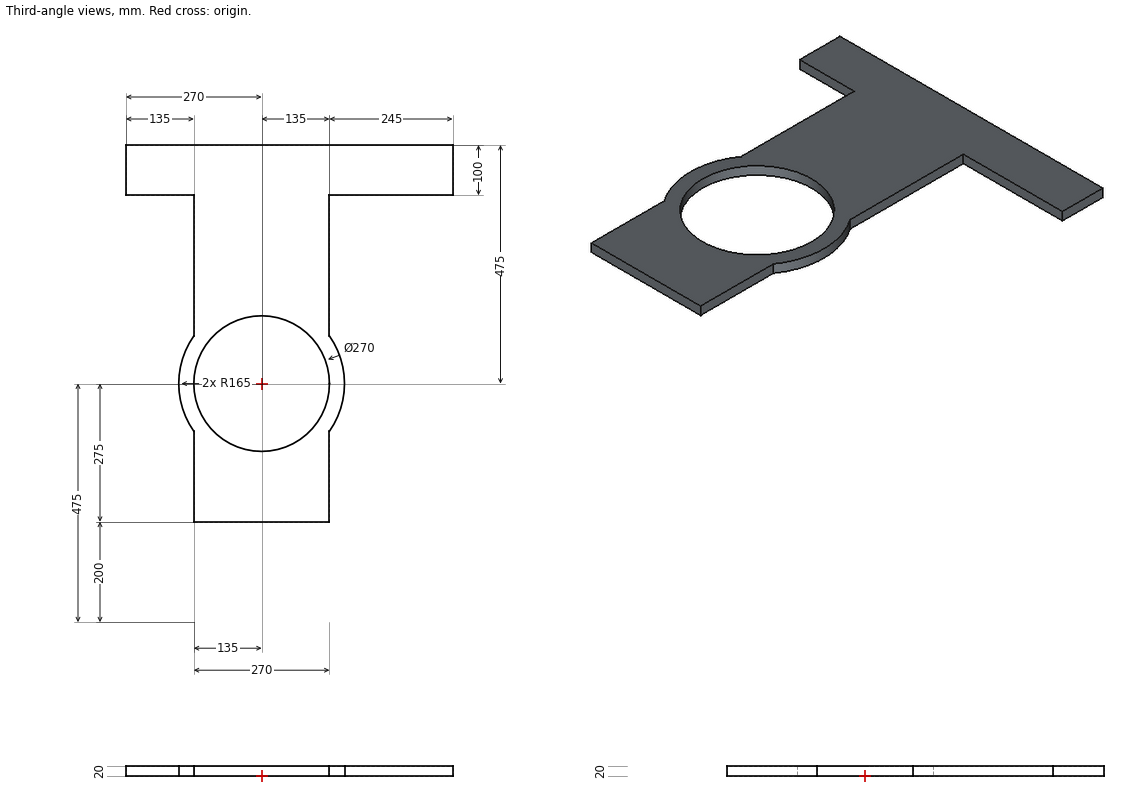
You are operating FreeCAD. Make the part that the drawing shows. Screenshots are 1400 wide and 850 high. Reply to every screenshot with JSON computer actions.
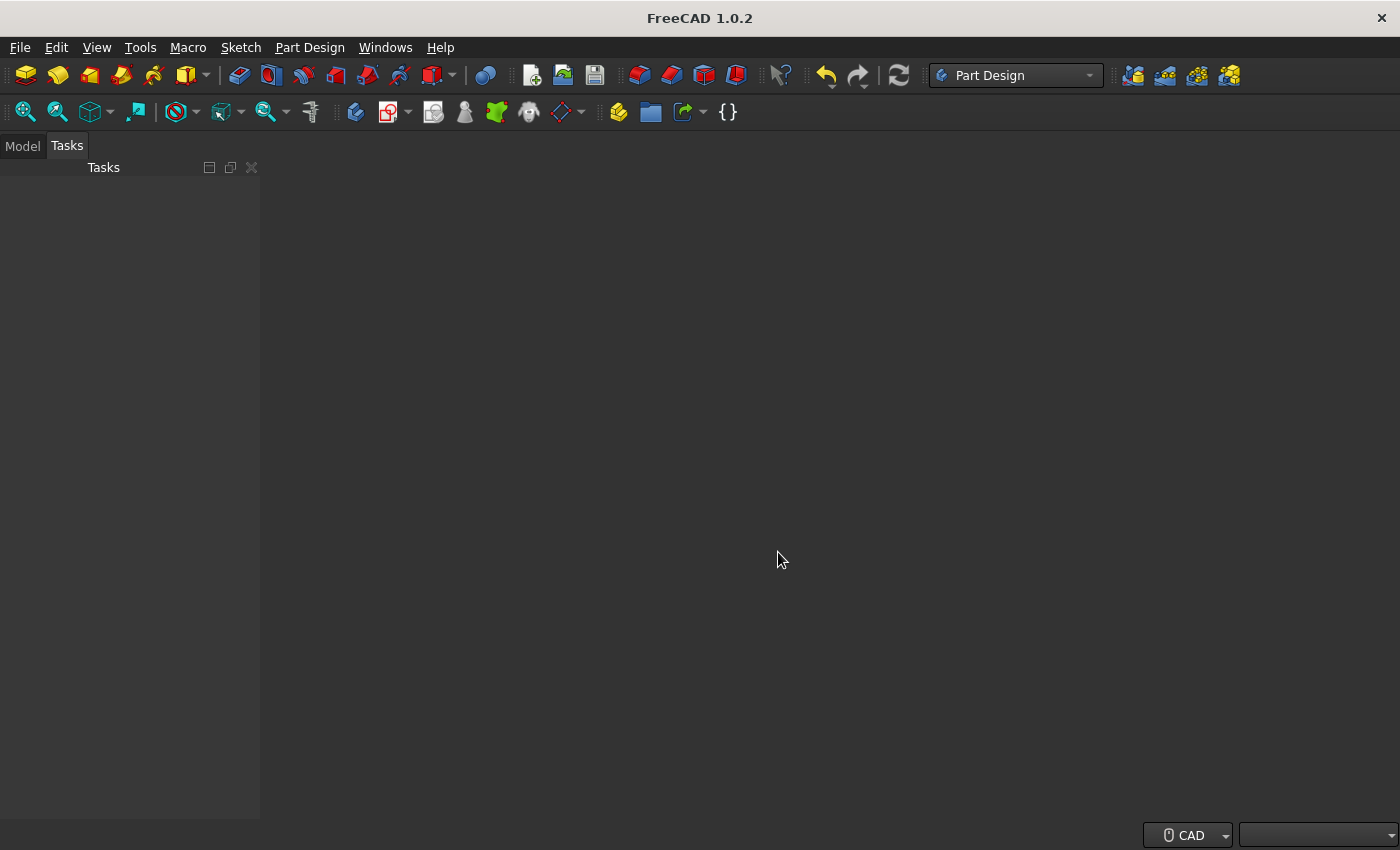
{"action": "key", "text": "ctrl+n"}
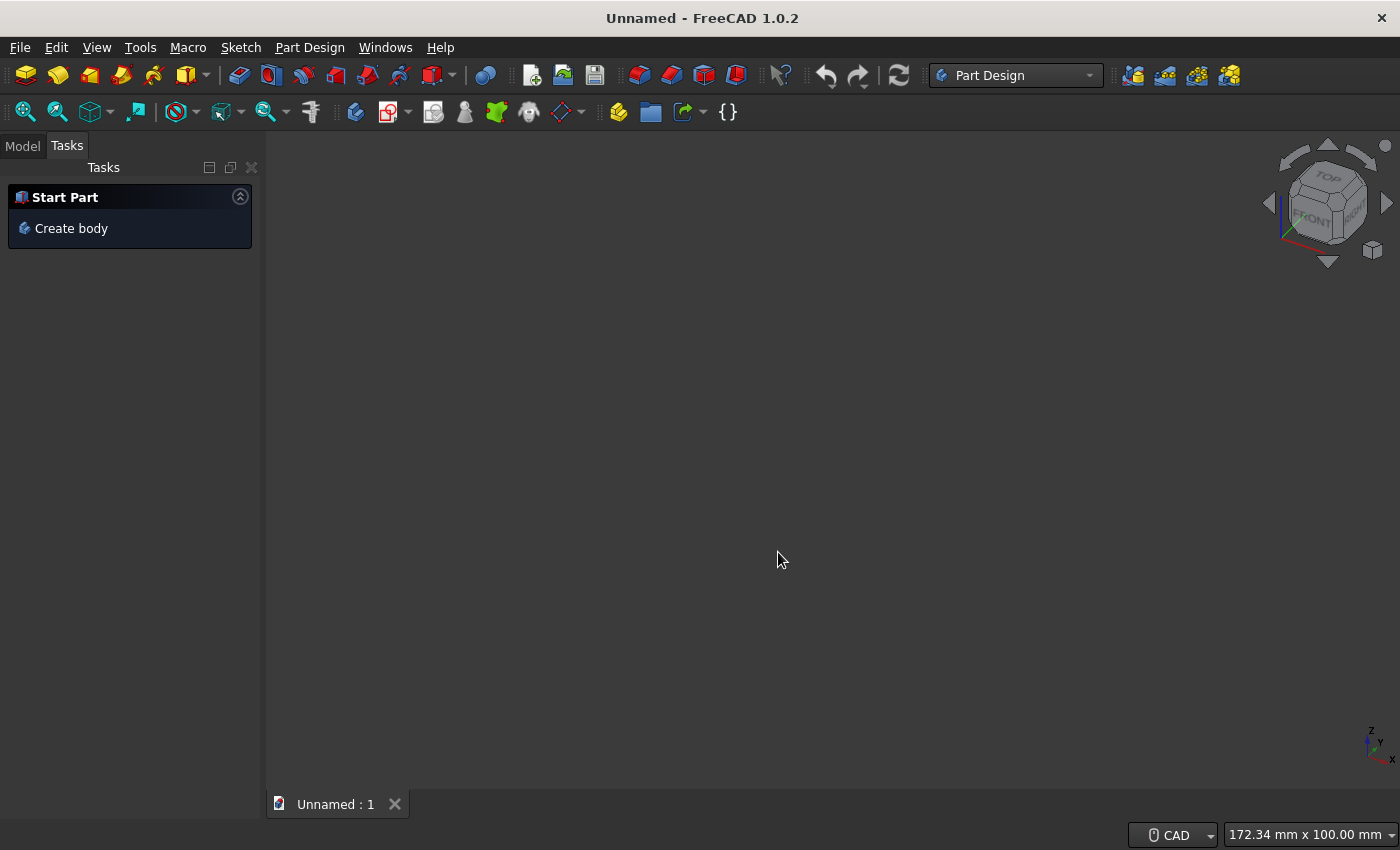
{"action": "left_click", "coordinate": [388, 112]}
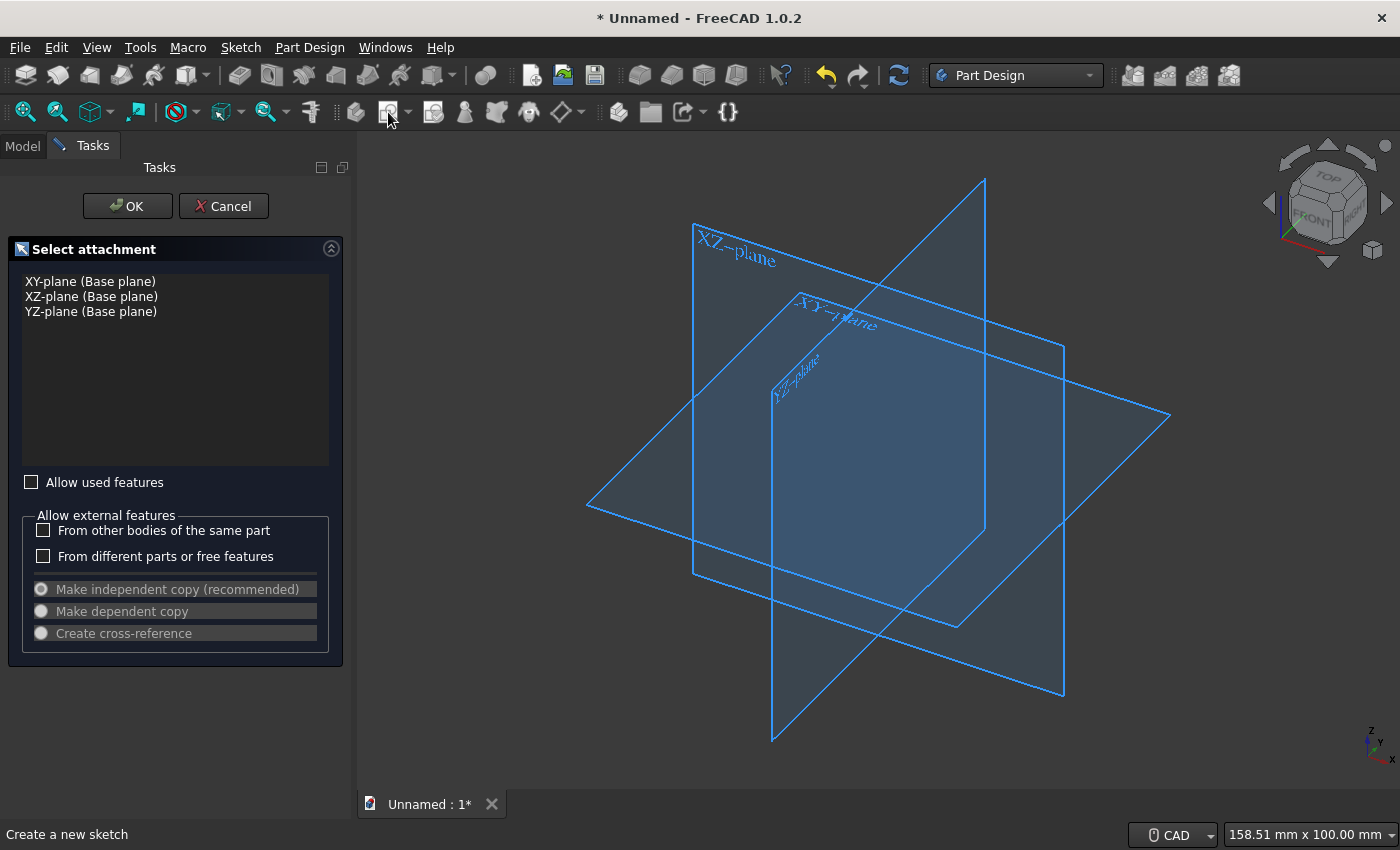
{"action": "left_click", "coordinate": [82, 282]}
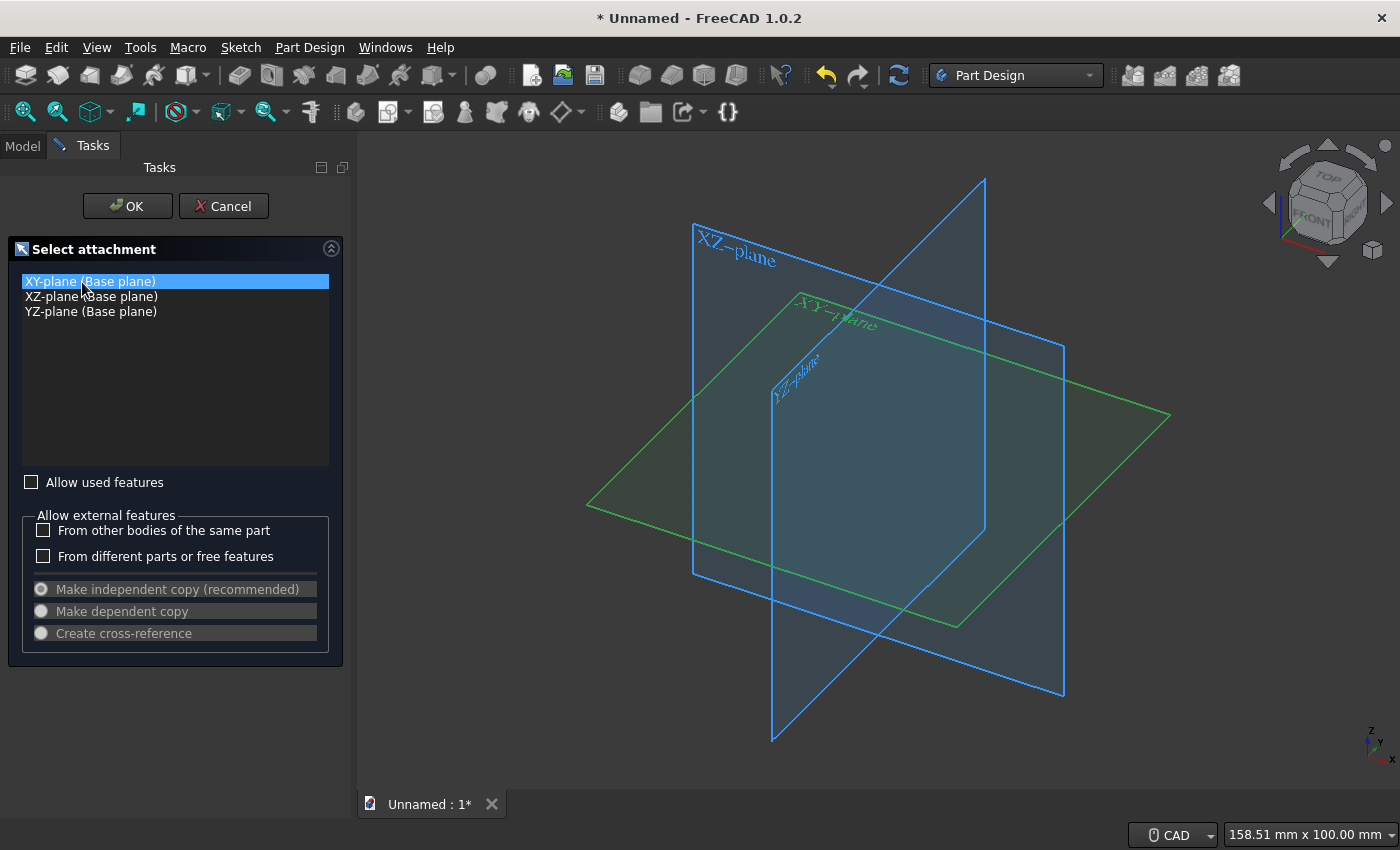
{"action": "left_click", "coordinate": [128, 206]}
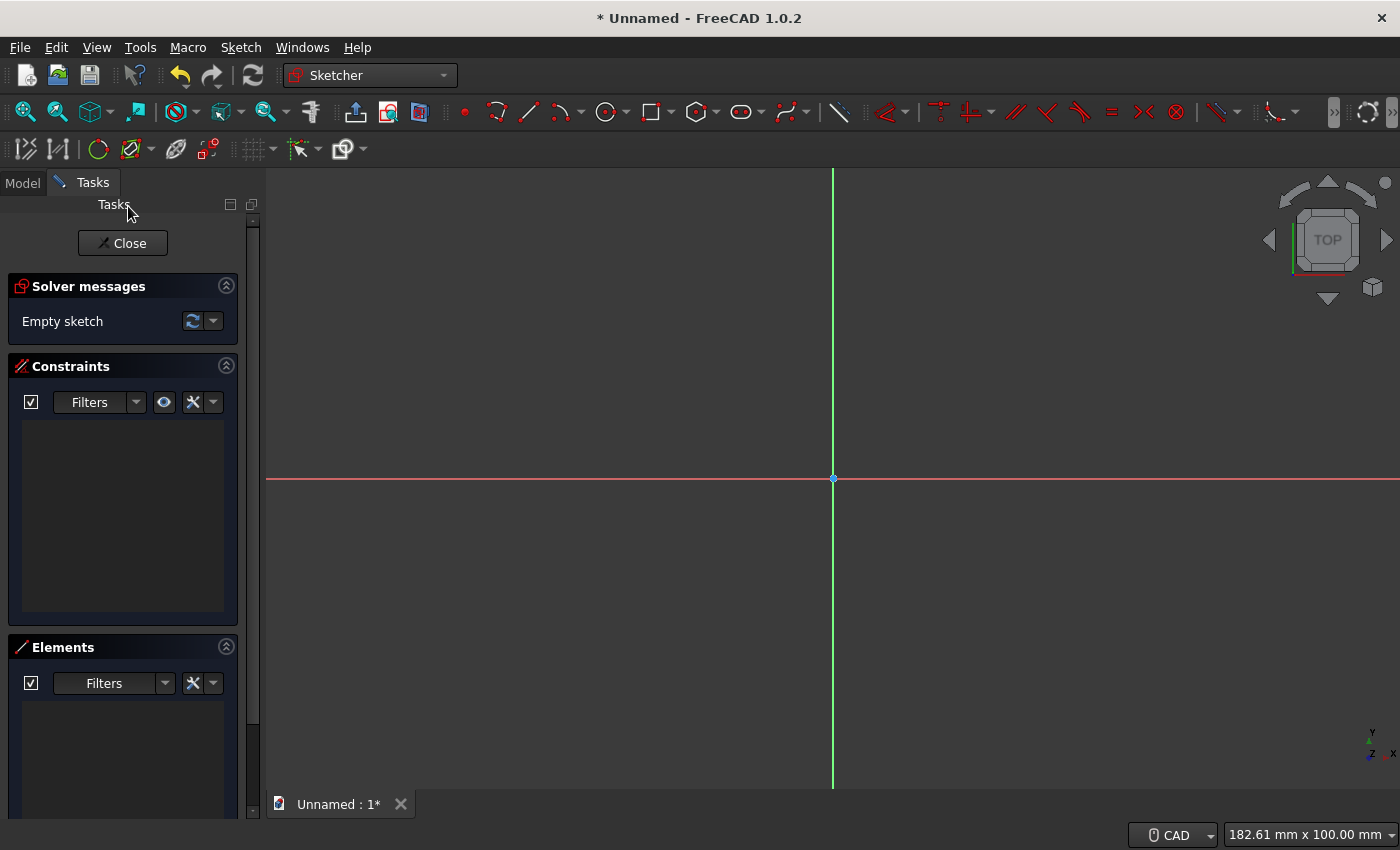
{"action": "scroll", "coordinate": [759, 478], "scroll_direction": "down", "scroll_amount": 13}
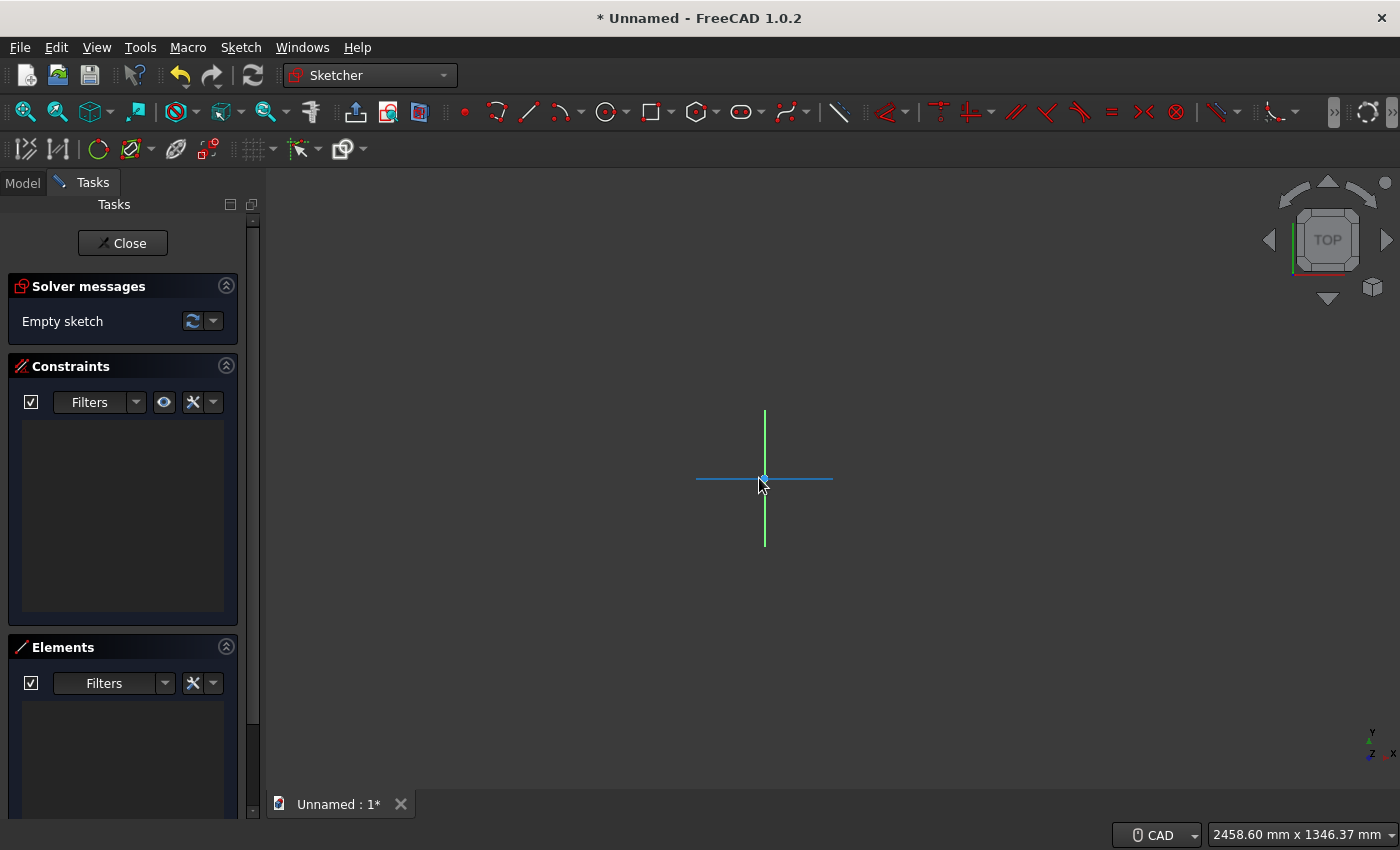
{"action": "key", "text": "g m"}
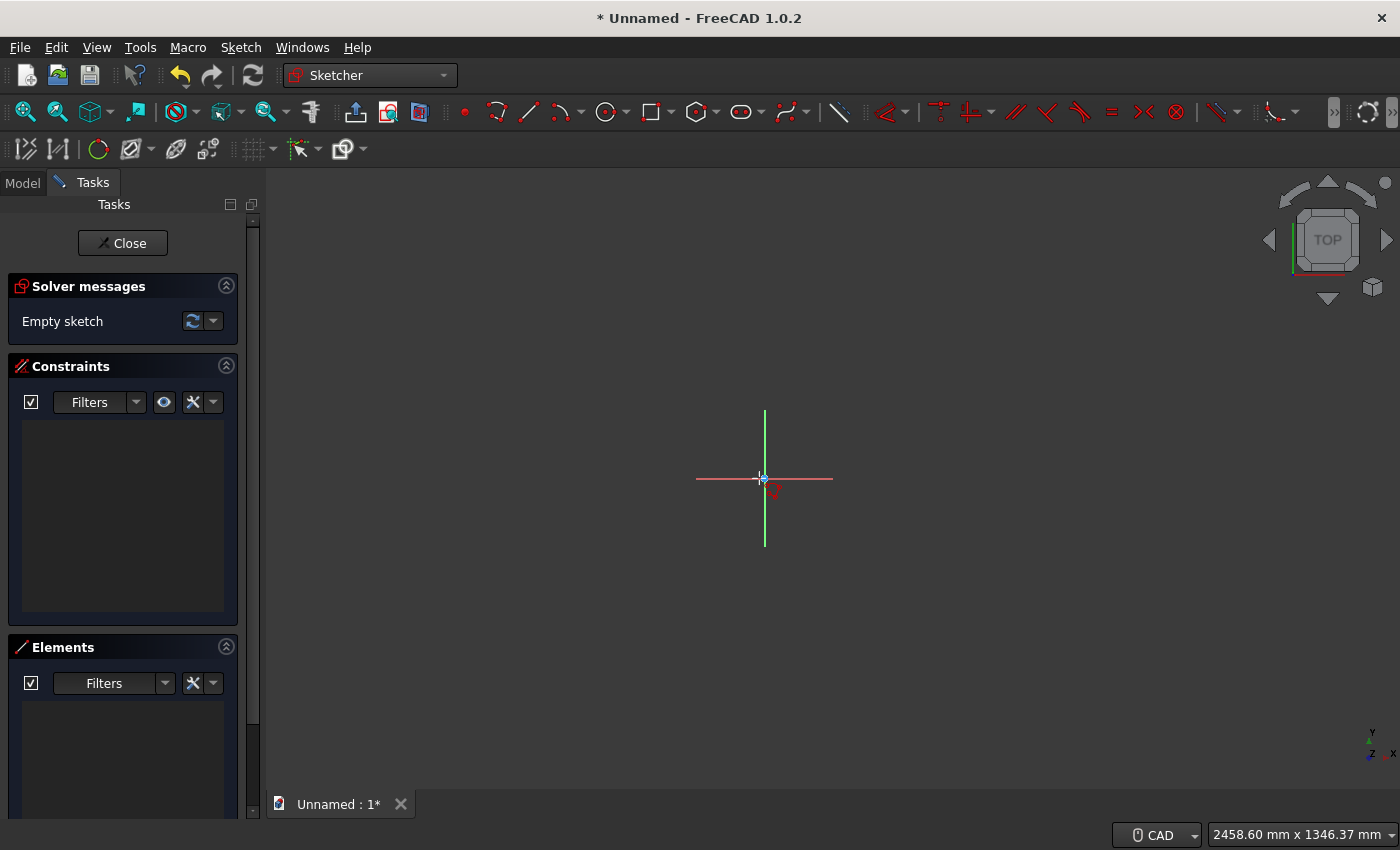
{"action": "left_click", "coordinate": [703, 522]}
{"action": "left_click", "coordinate": [703, 698]}
{"action": "left_click", "coordinate": [827, 698]}
{"action": "left_click", "coordinate": [827, 522]}
{"action": "right_click", "coordinate": [827, 522]}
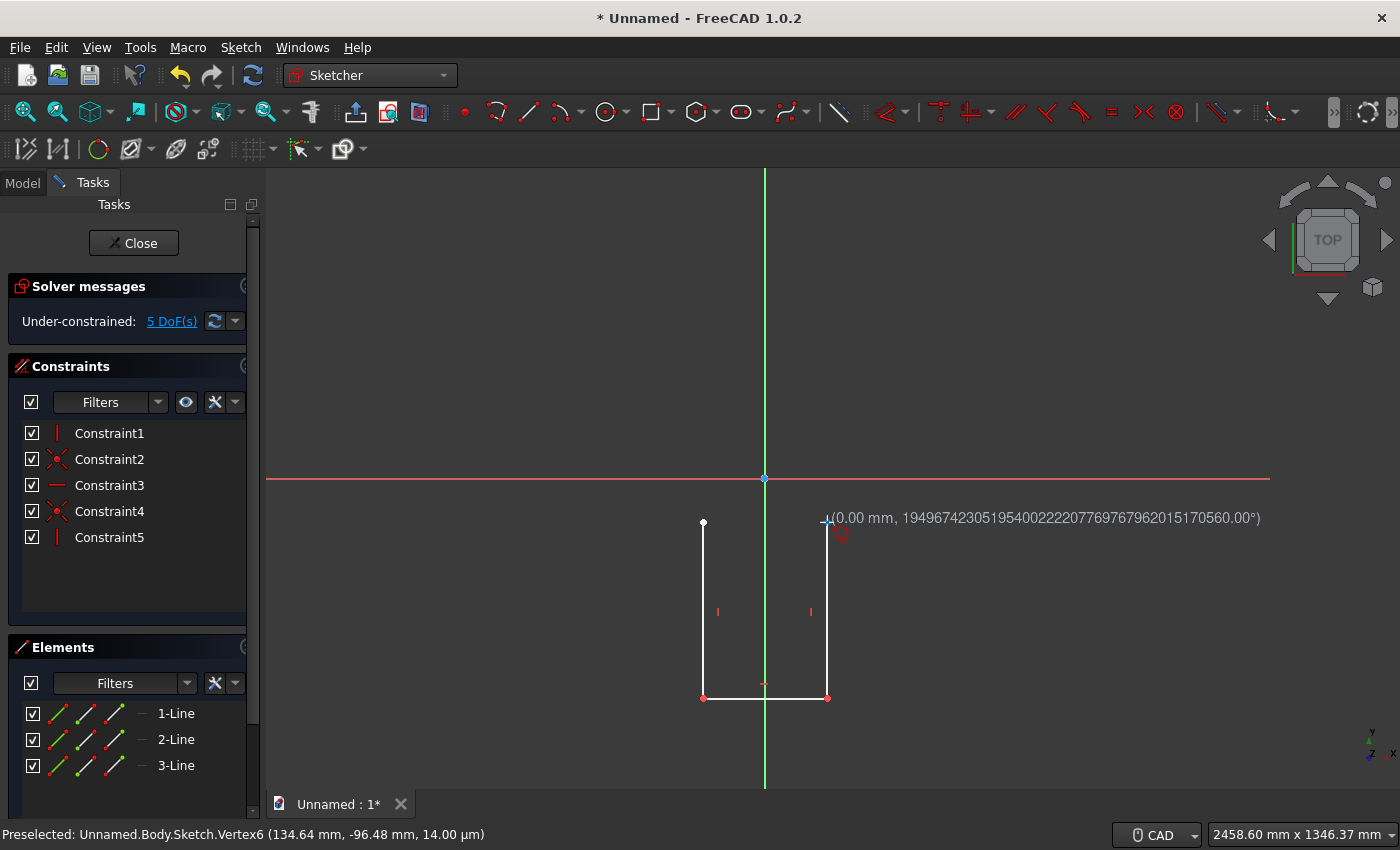
{"action": "left_click", "coordinate": [827, 435]}
{"action": "left_click", "coordinate": [827, 259]}
{"action": "left_click", "coordinate": [703, 259]}
{"action": "left_click", "coordinate": [703, 435]}
{"action": "right_click", "coordinate": [703, 435]}